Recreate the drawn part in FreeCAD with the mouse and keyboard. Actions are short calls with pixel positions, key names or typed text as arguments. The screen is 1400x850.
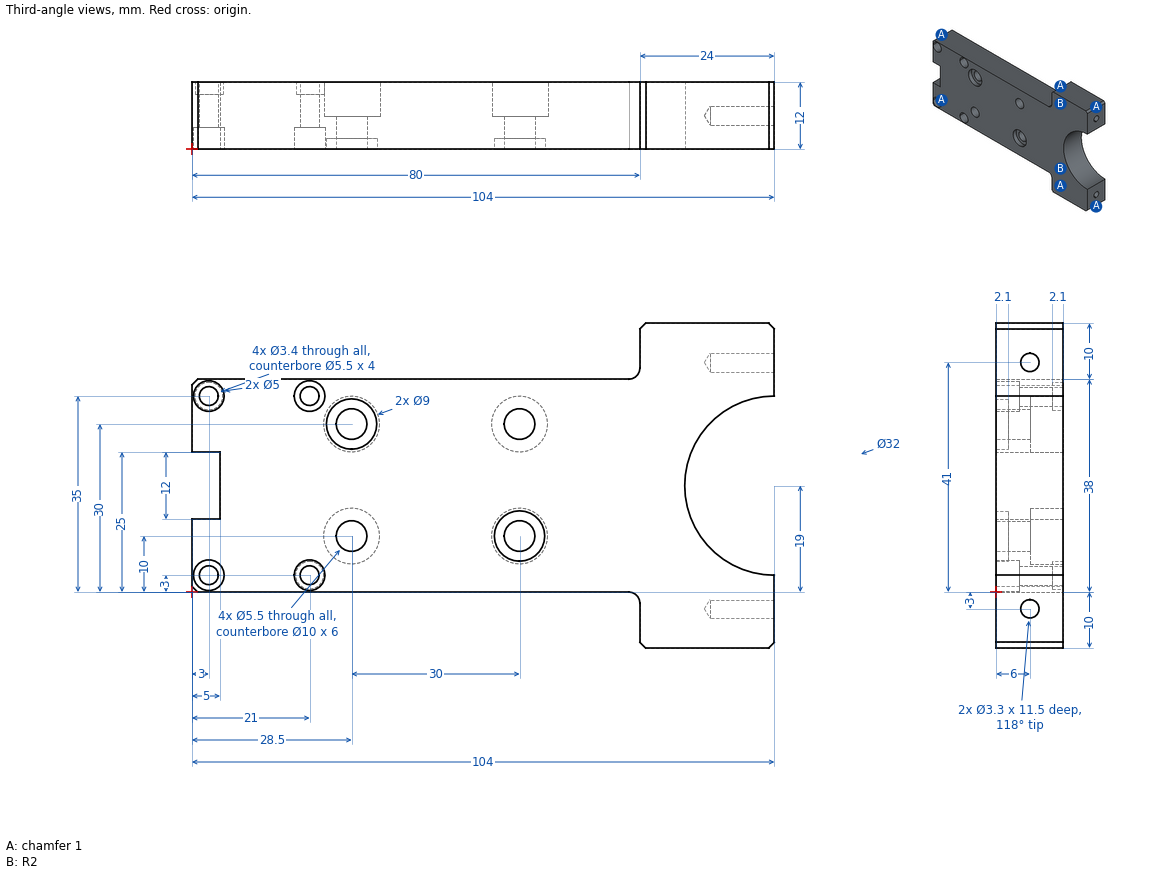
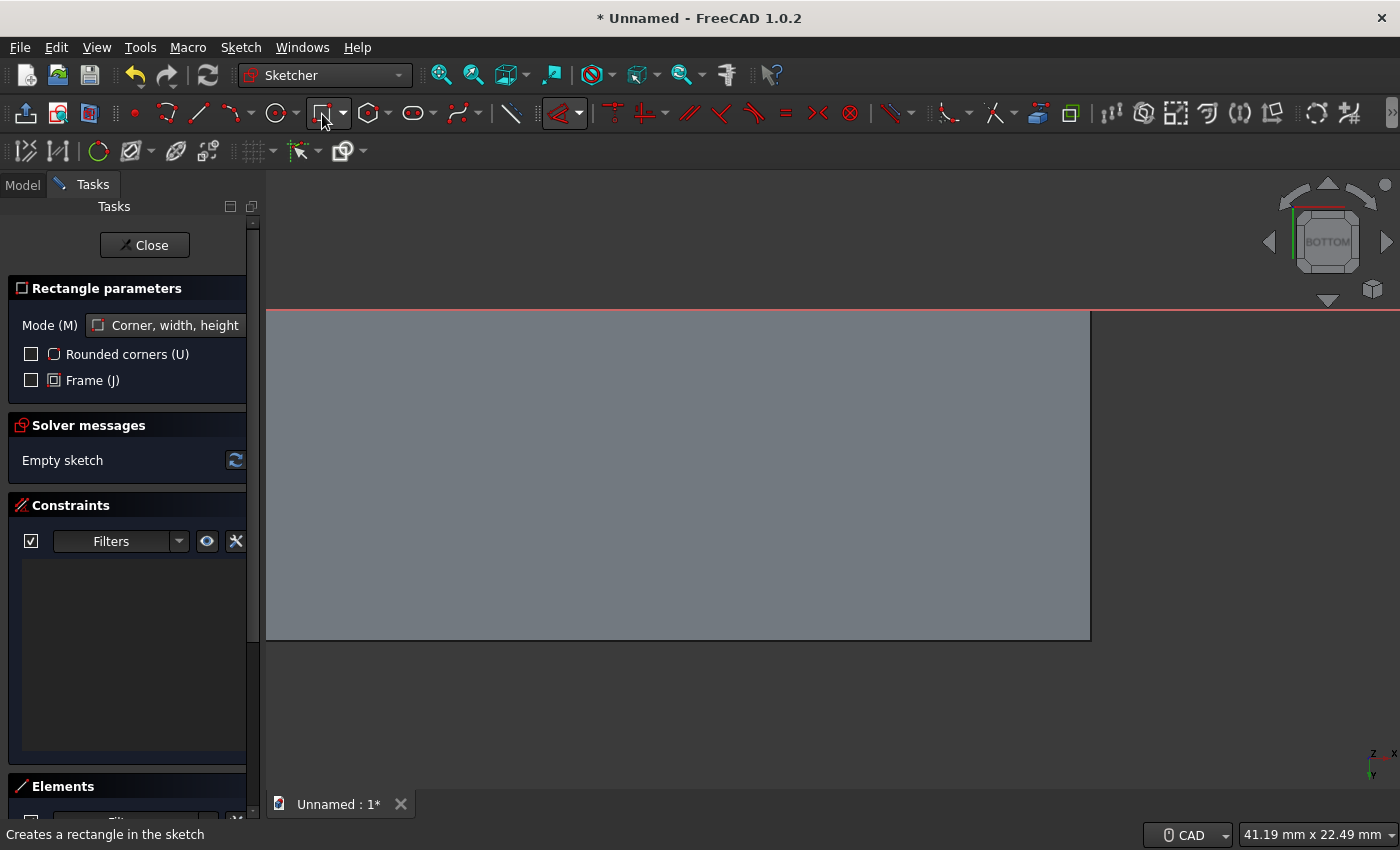
click(431, 310)
click(1091, 641)
key(Escape)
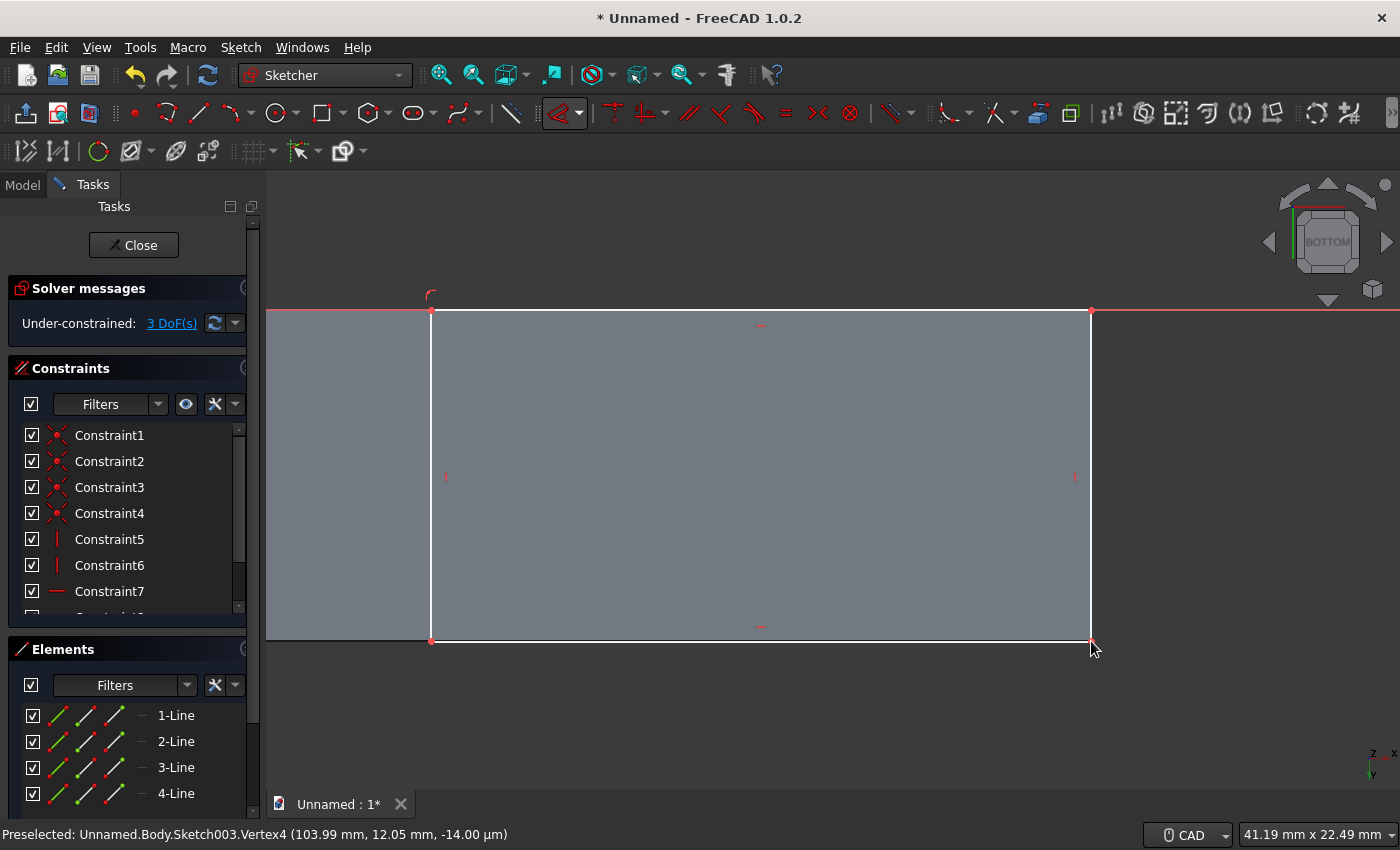
click(431, 410)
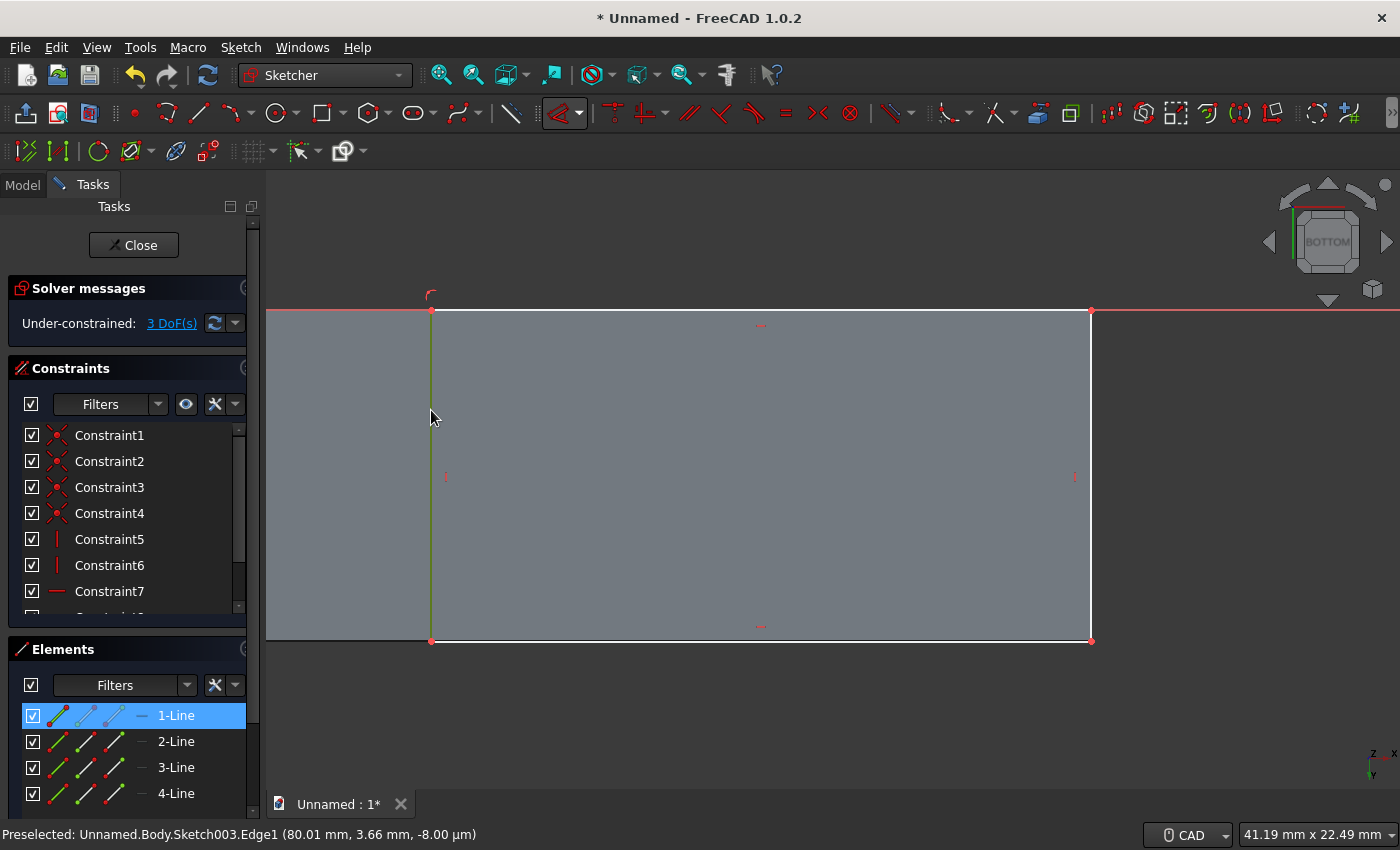
click(582, 114)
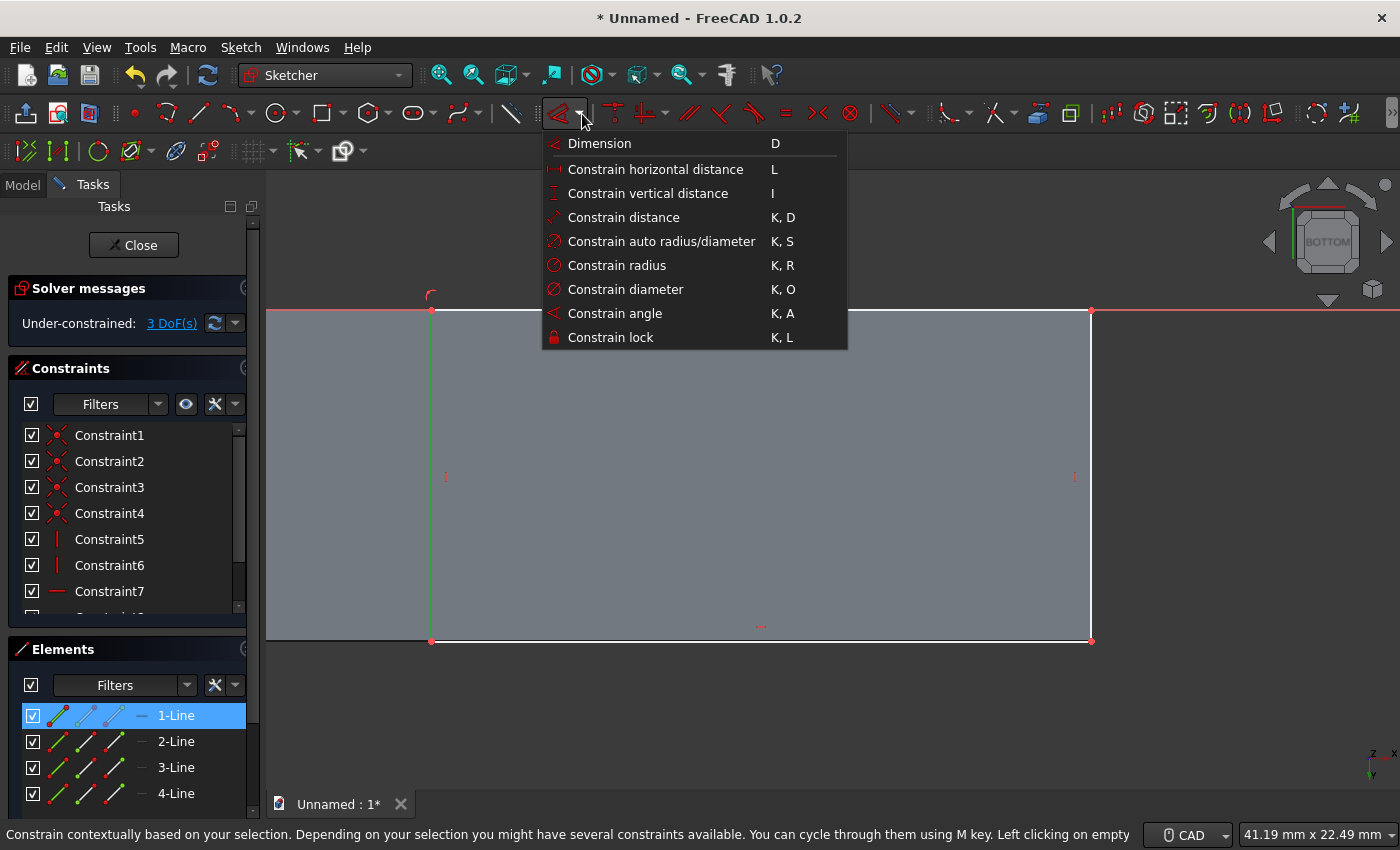
click(695, 193)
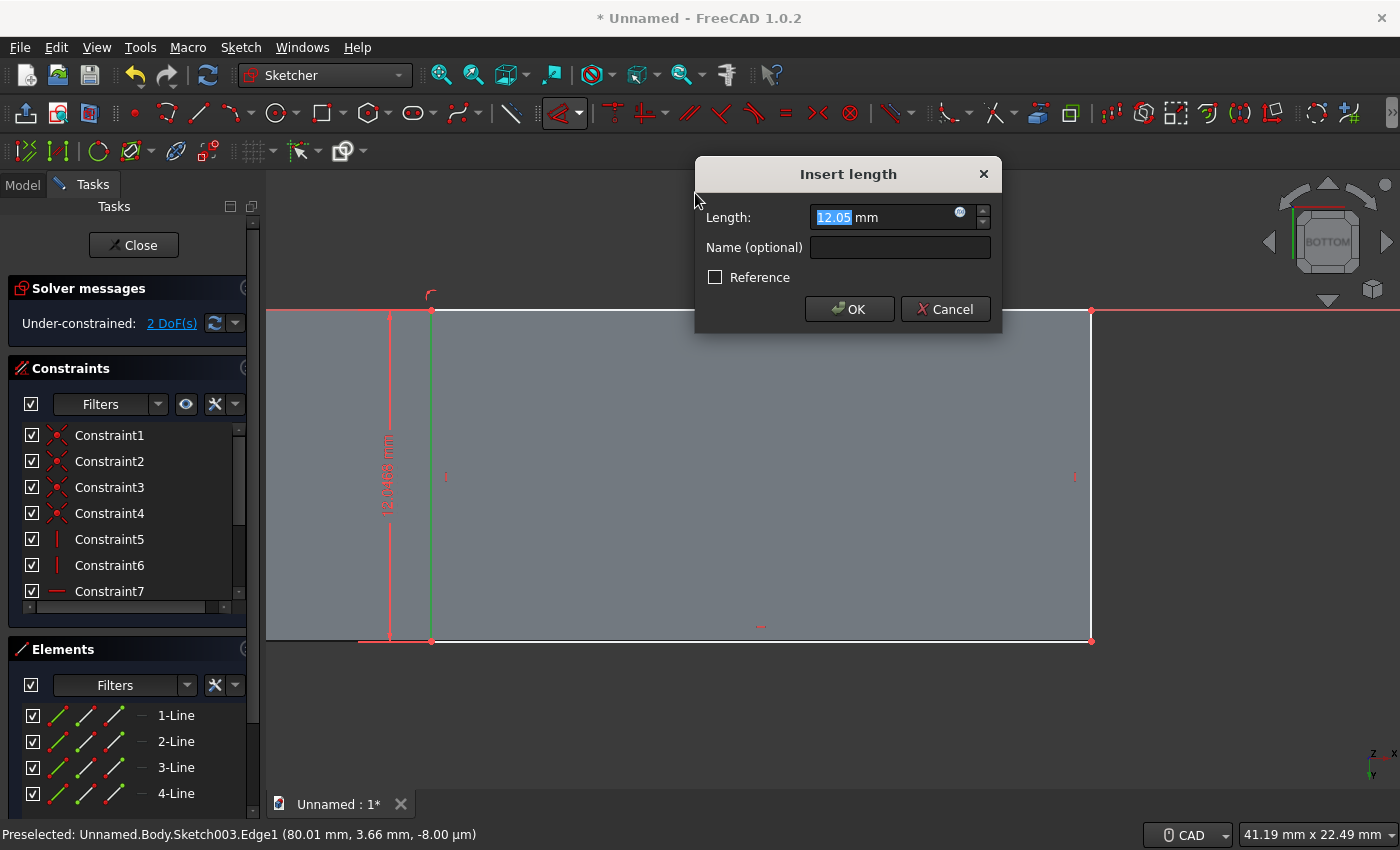
text(12)
key(Return)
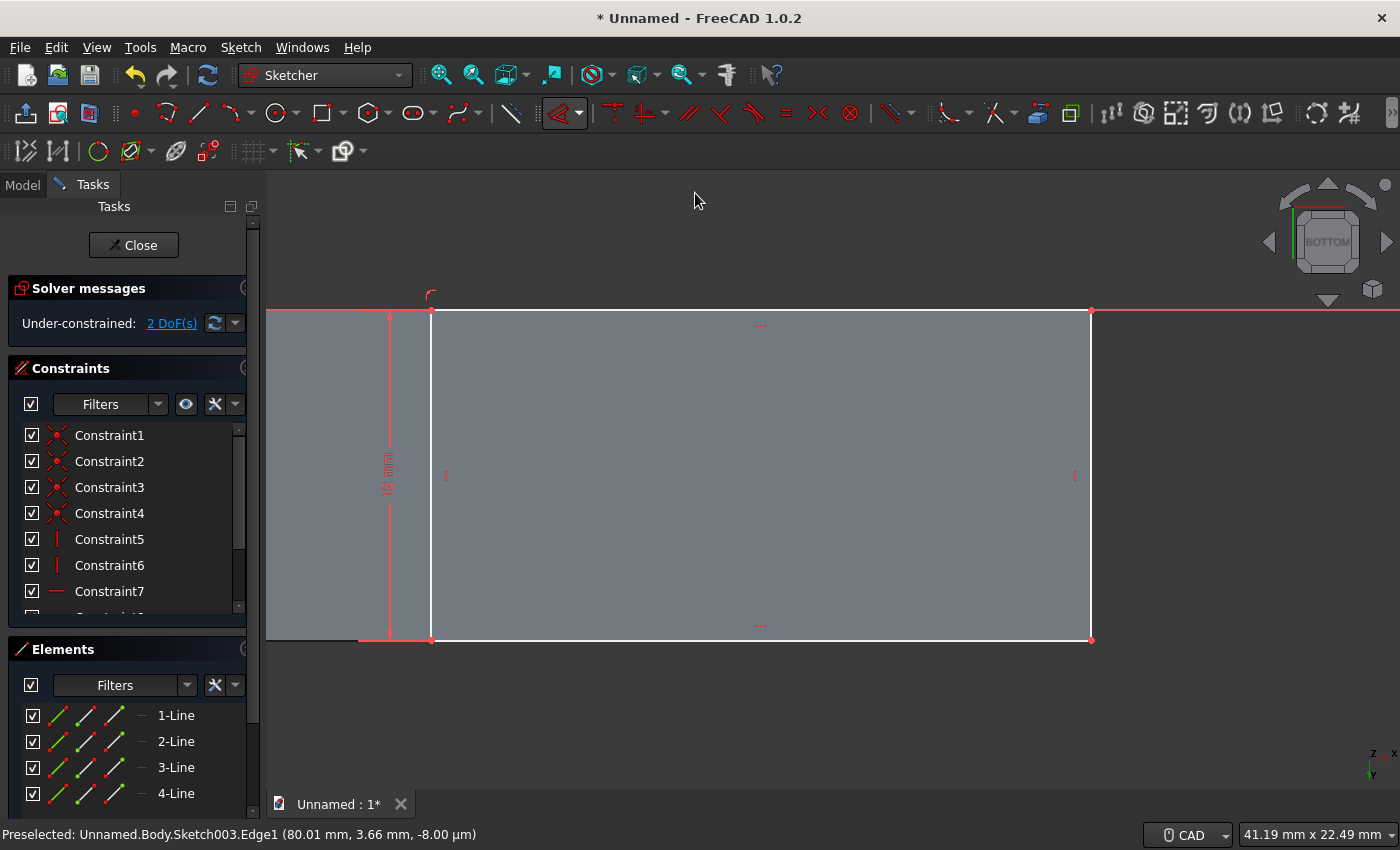
click(629, 641)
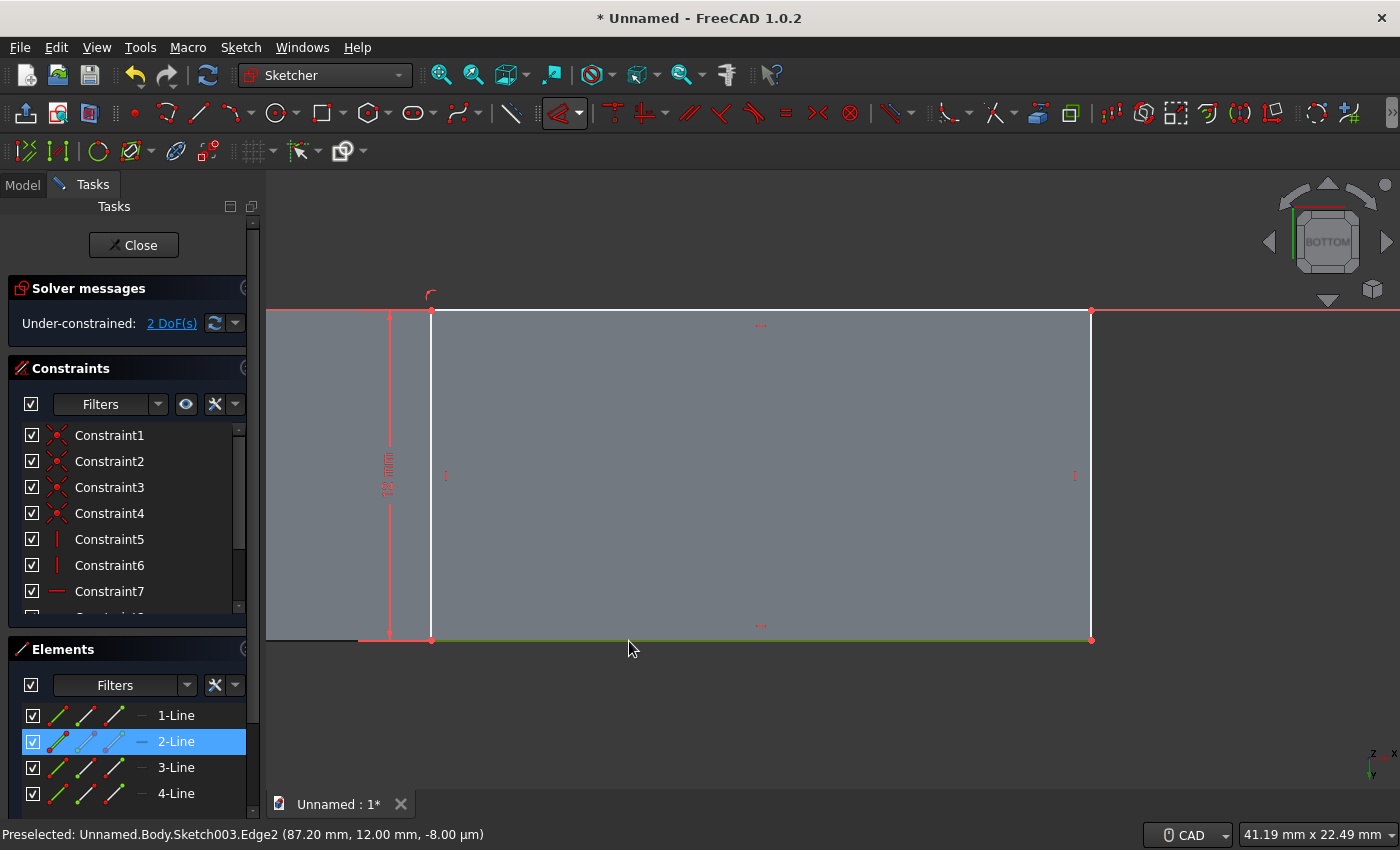
click(582, 114)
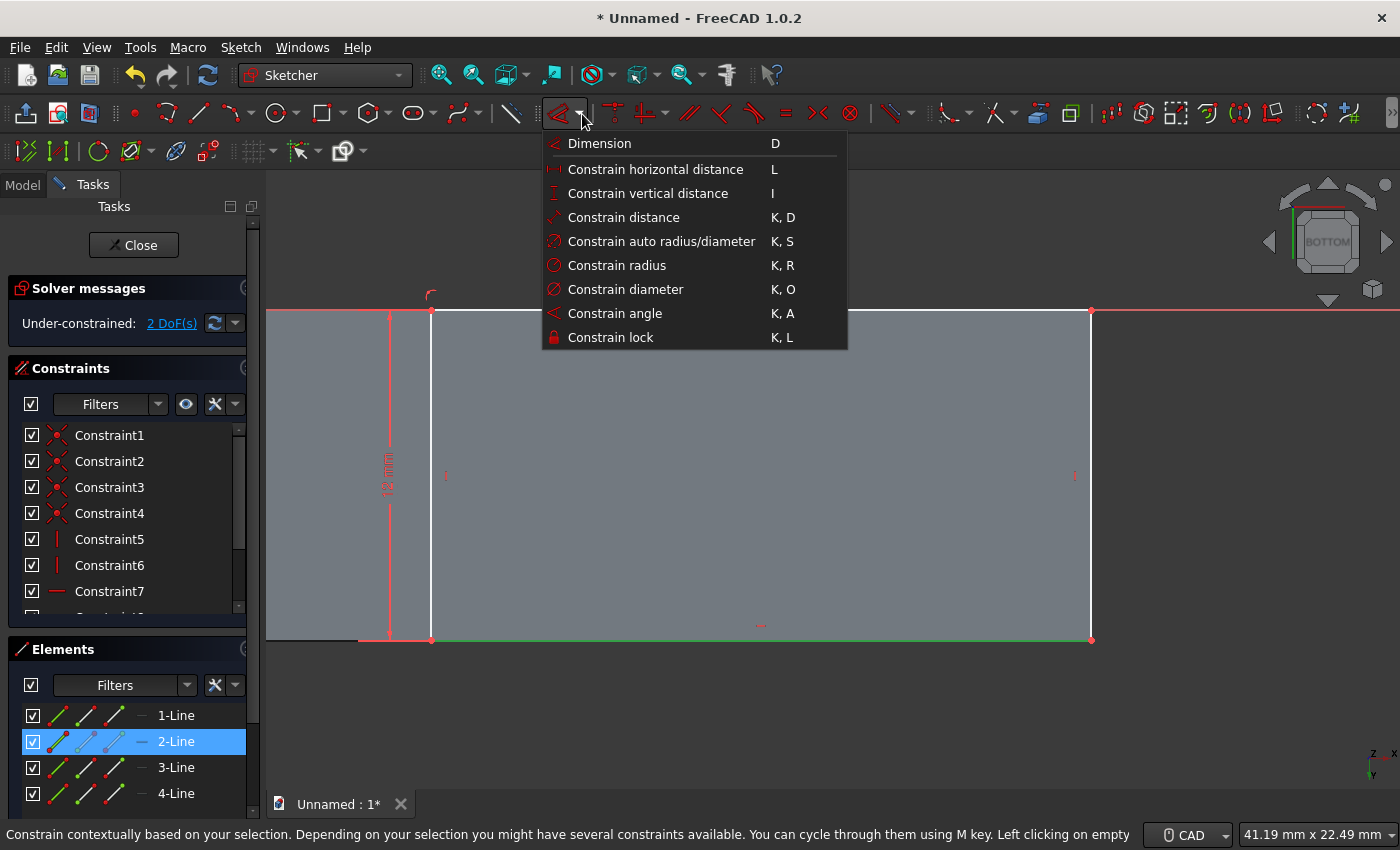
click(695, 169)